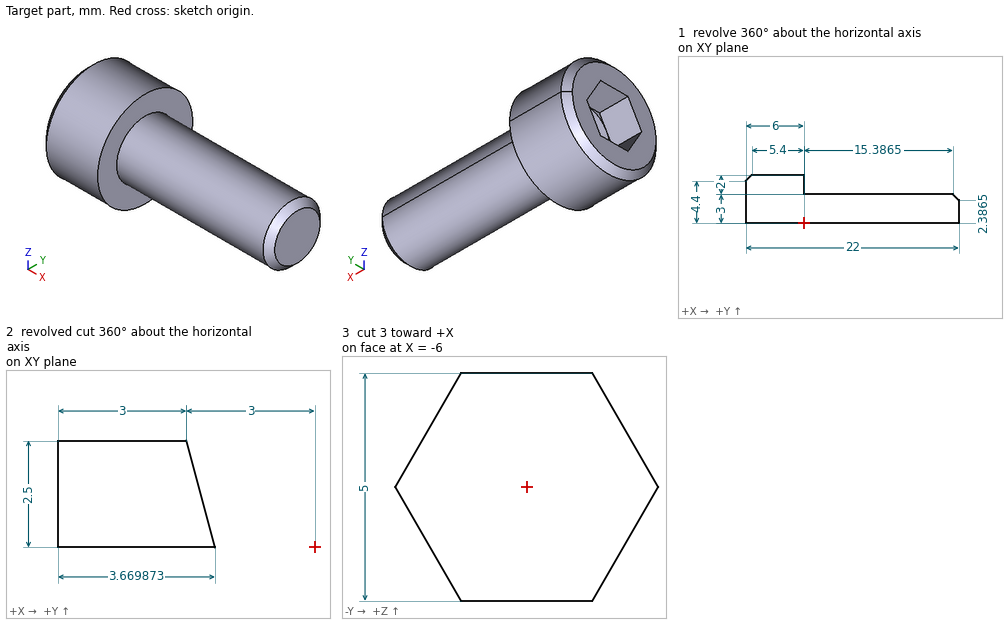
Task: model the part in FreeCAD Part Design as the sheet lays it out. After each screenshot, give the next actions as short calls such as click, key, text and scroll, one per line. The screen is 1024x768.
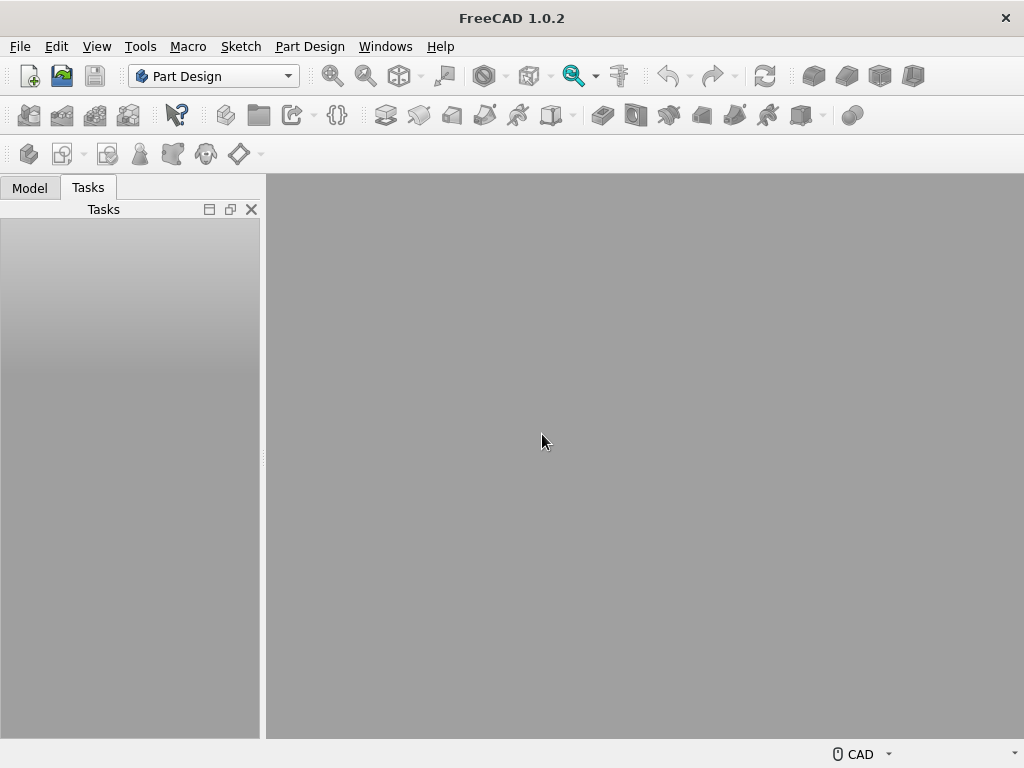
click(29, 76)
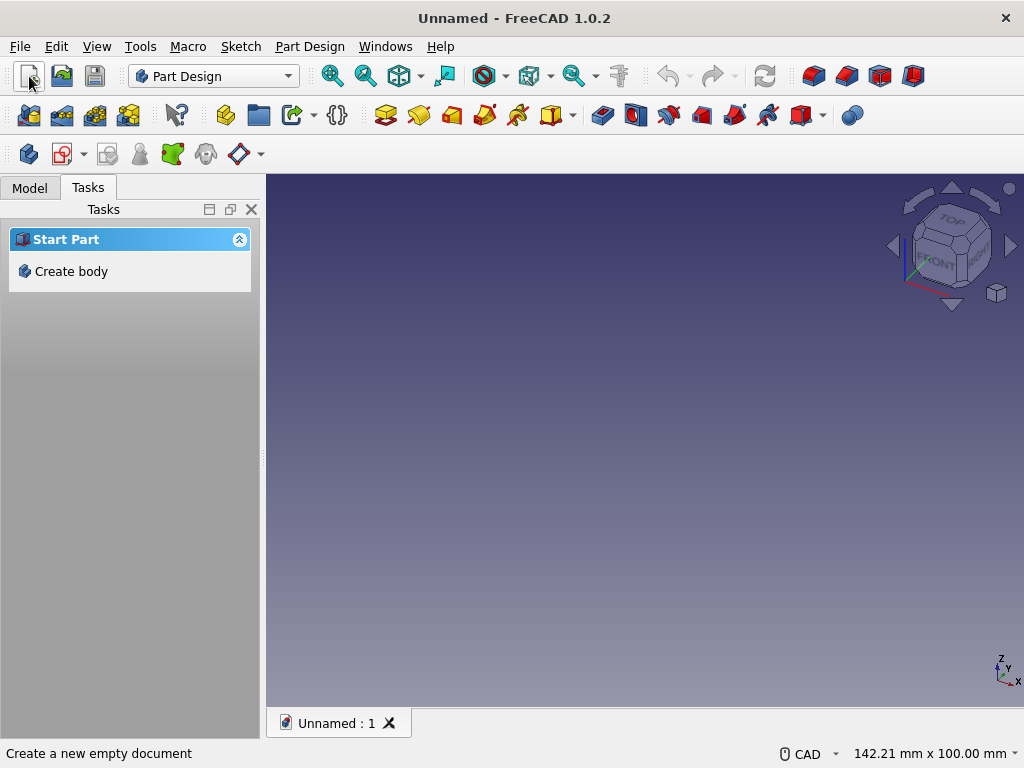
click(62, 154)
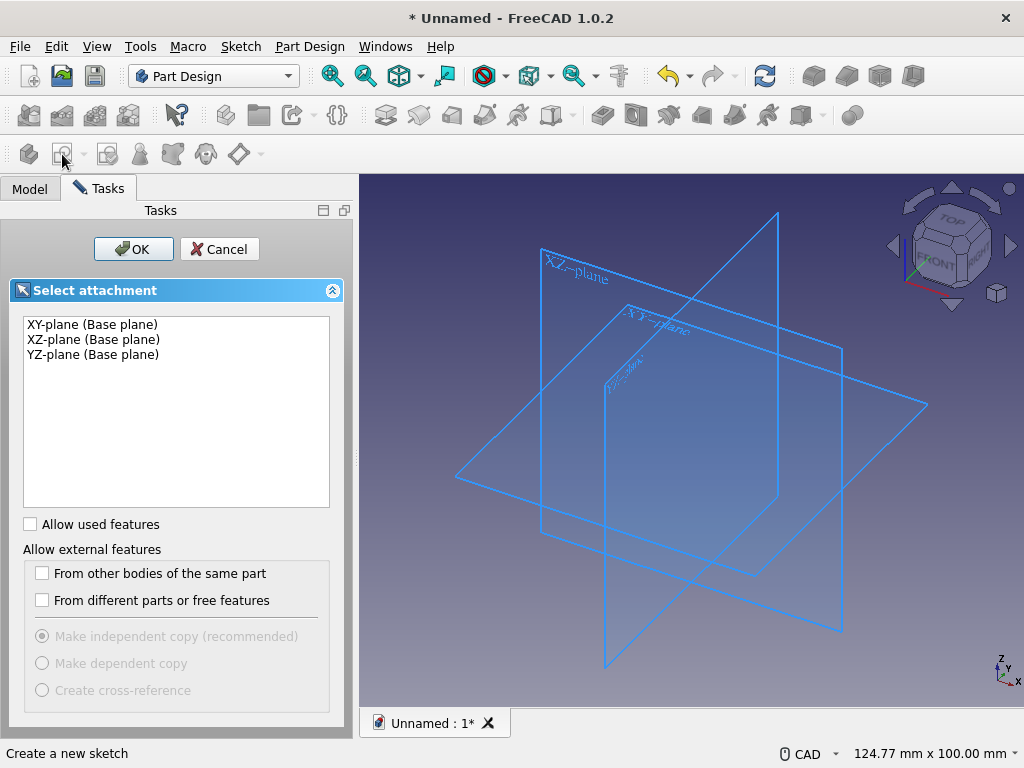
click(84, 324)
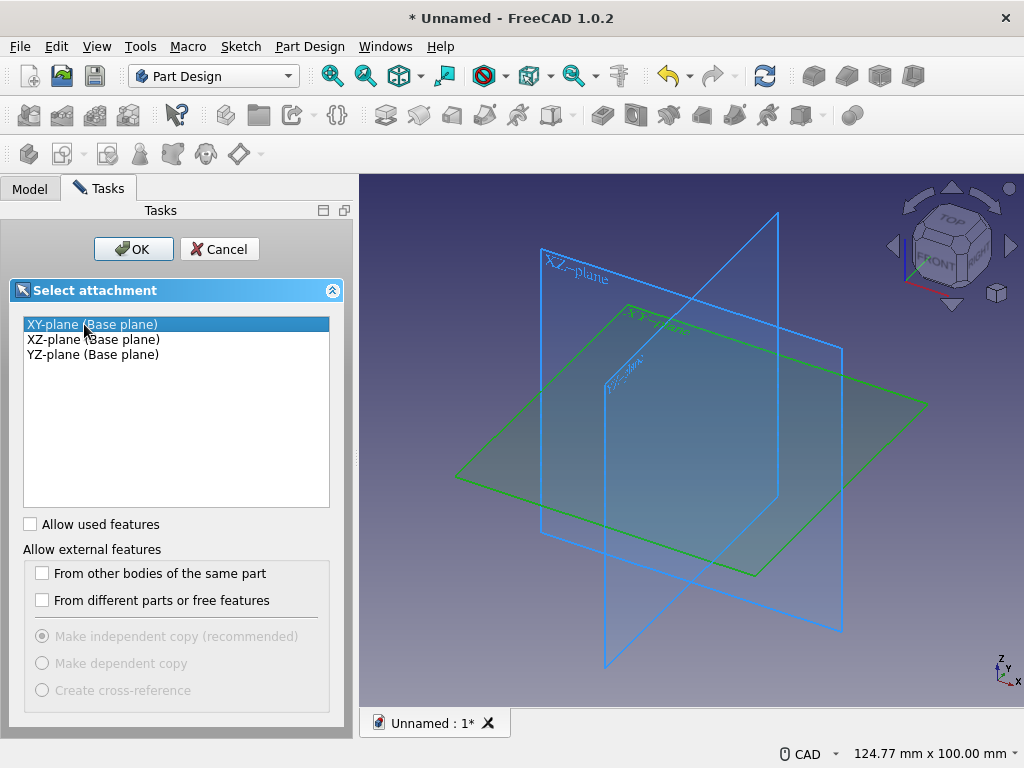
click(134, 249)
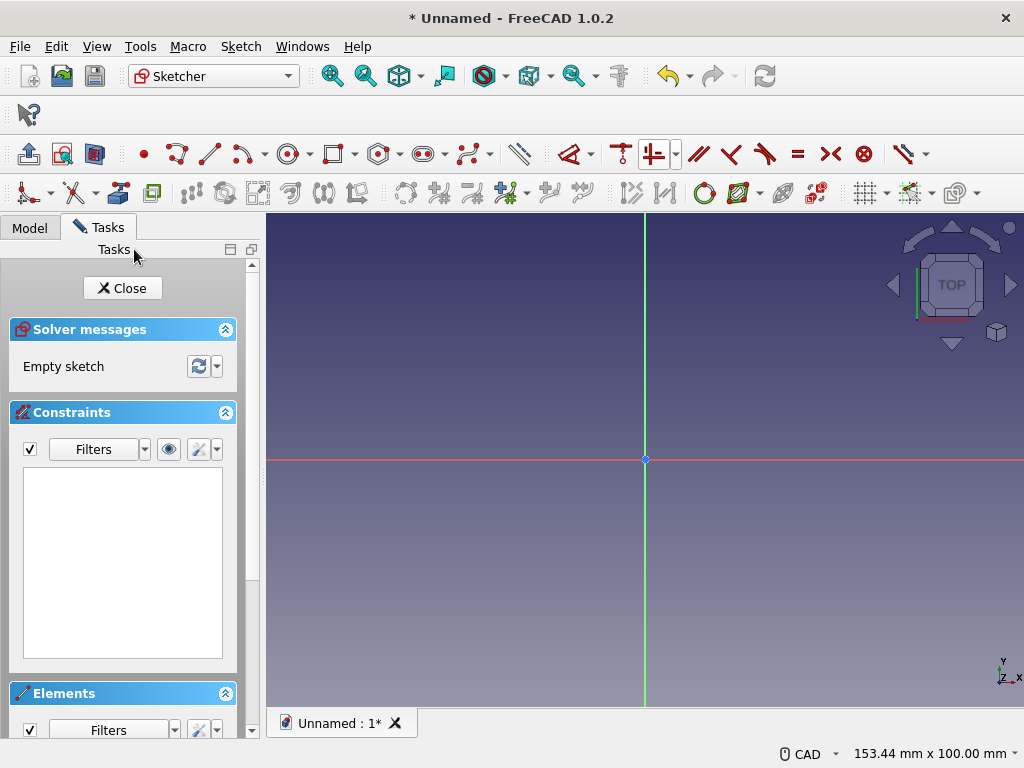
scroll(710, 442, up, 6)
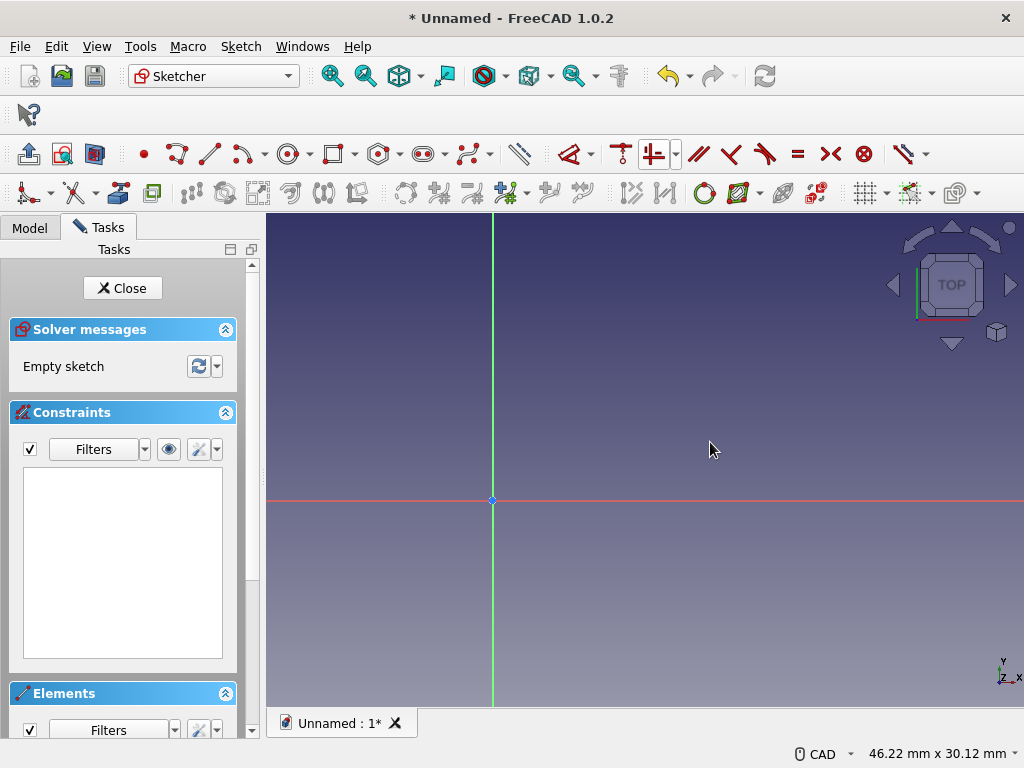
click(177, 154)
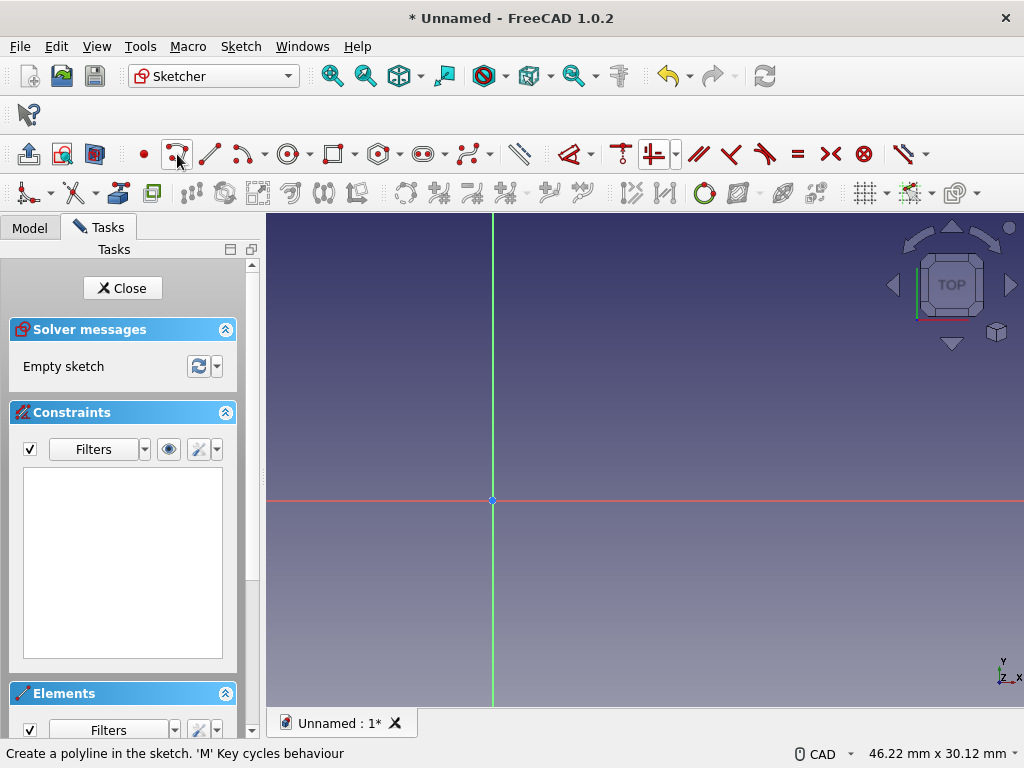
click(493, 451)
click(502, 419)
click(404, 419)
click(394, 429)
click(394, 501)
click(755, 492)
click(755, 462)
click(745, 451)
click(493, 452)
key(Escape)
key(Escape)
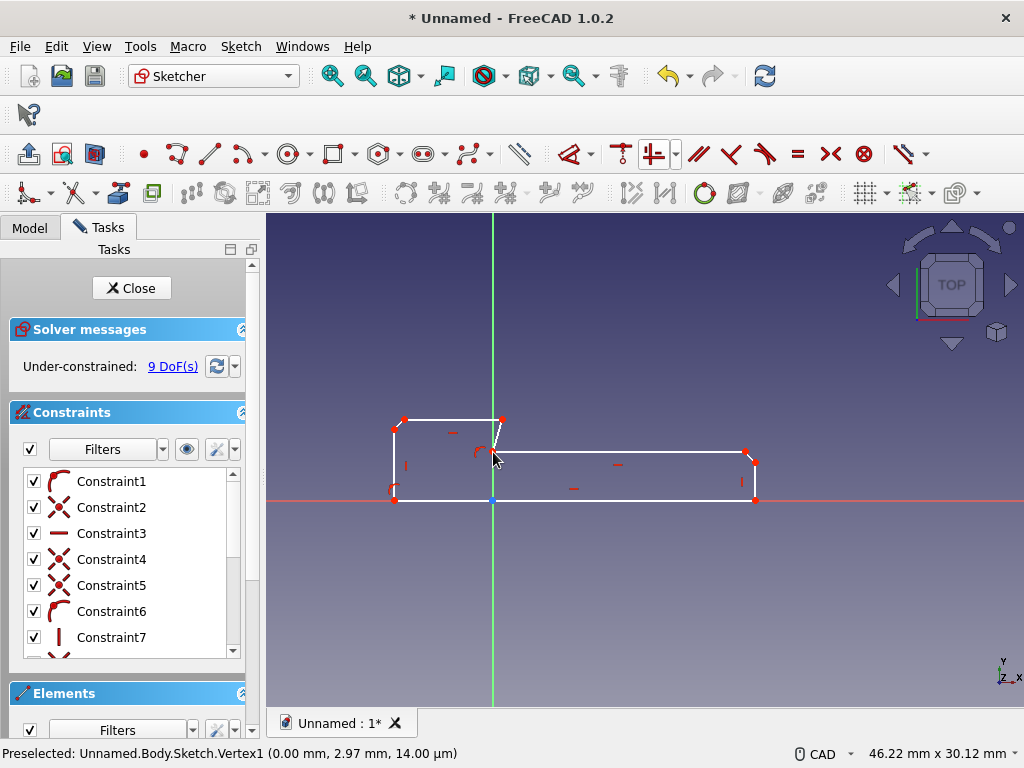
scroll(496, 442, up, 2)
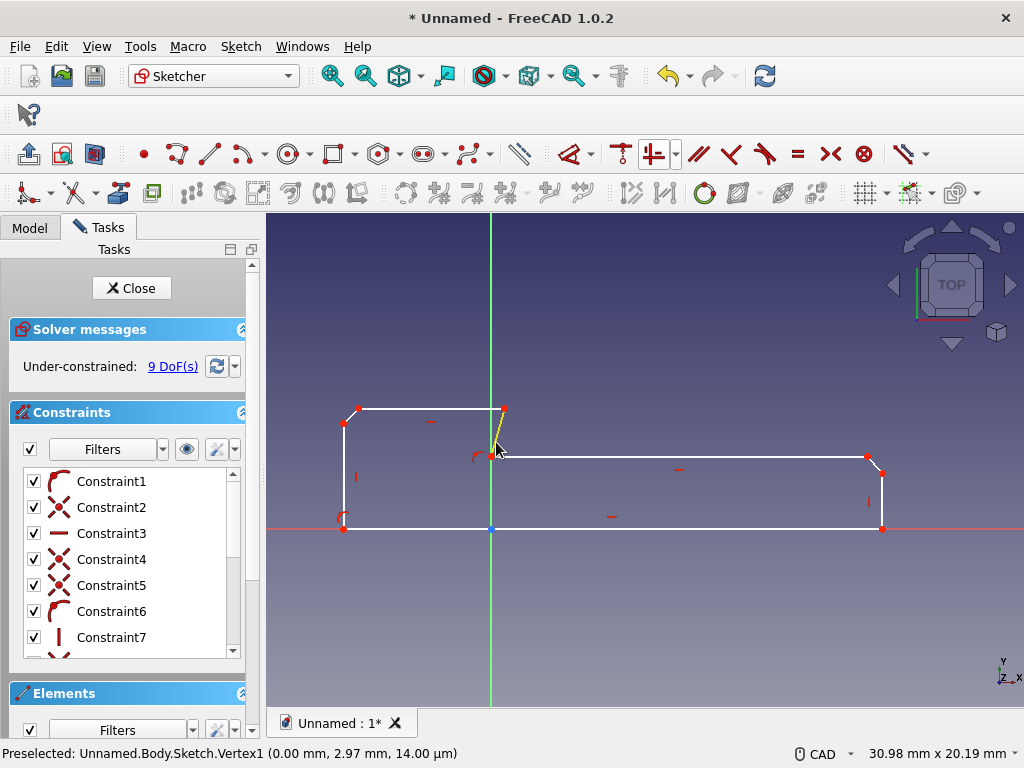
click(495, 442)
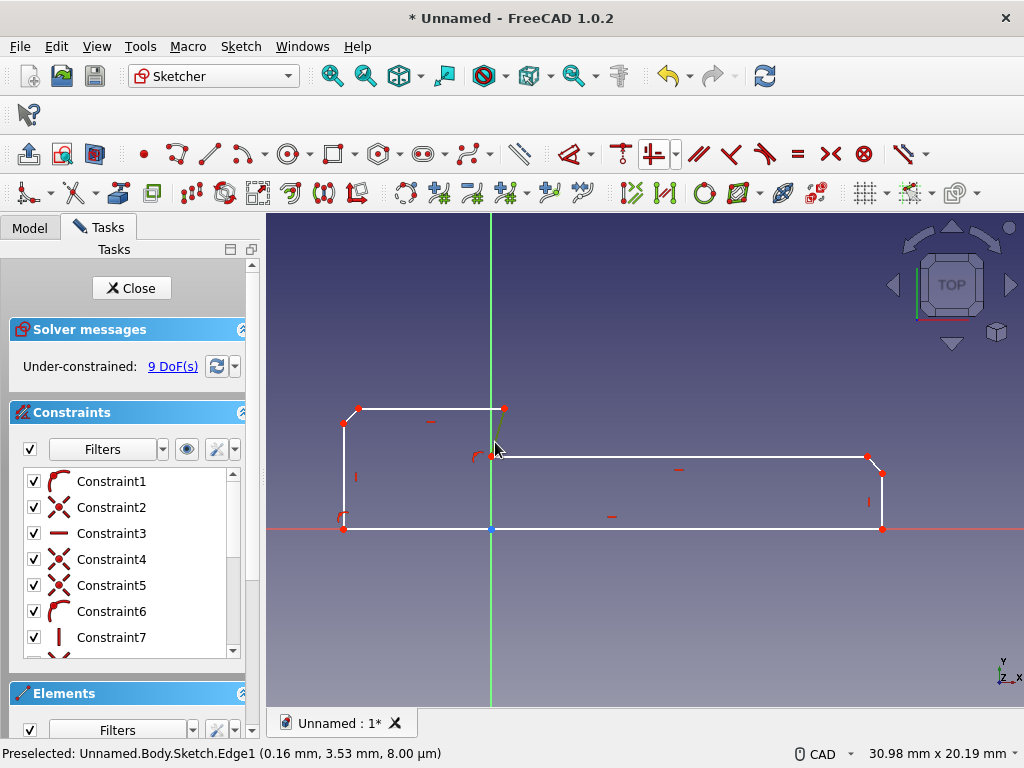
key(v)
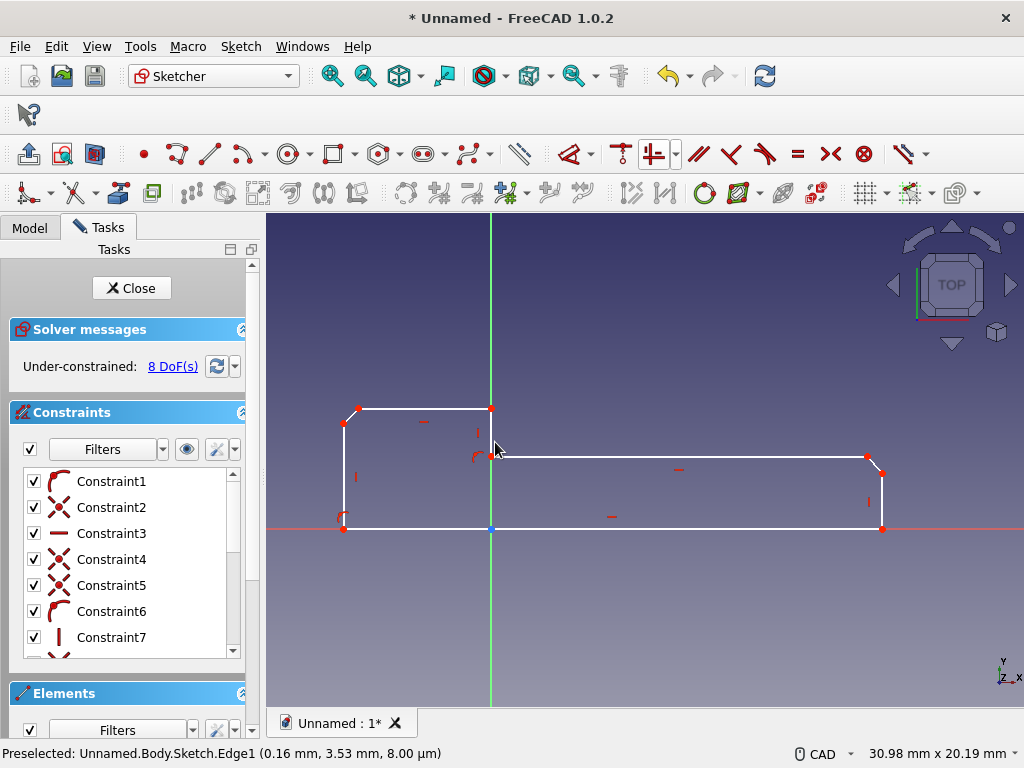
click(568, 154)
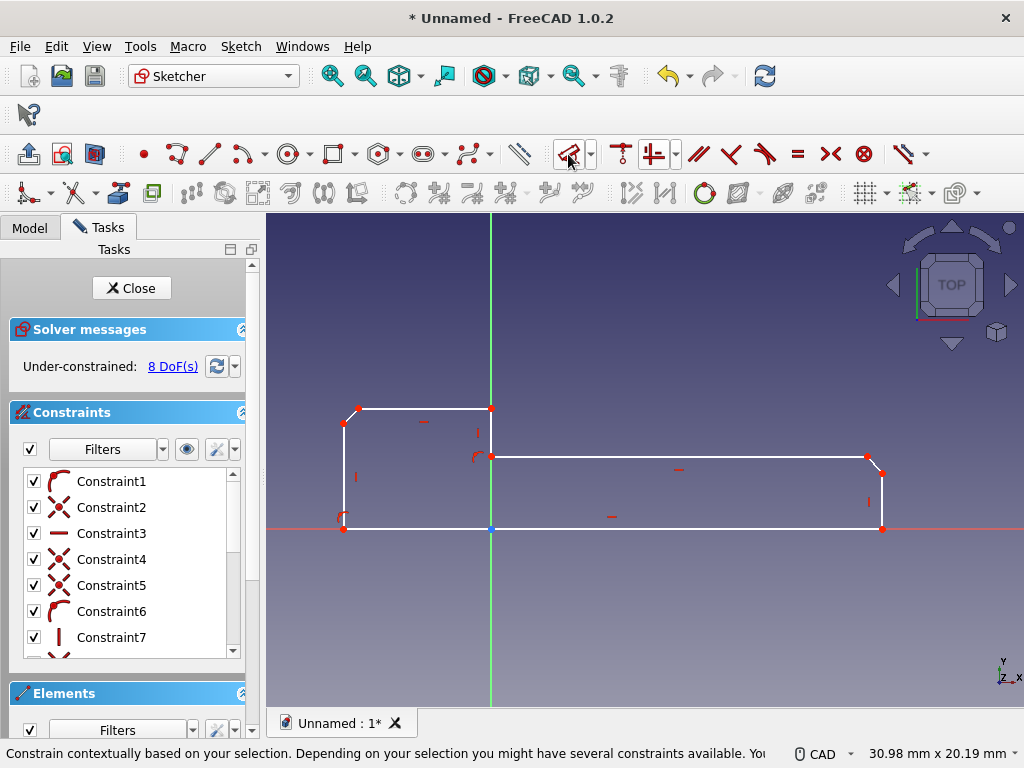
click(491, 442)
click(457, 433)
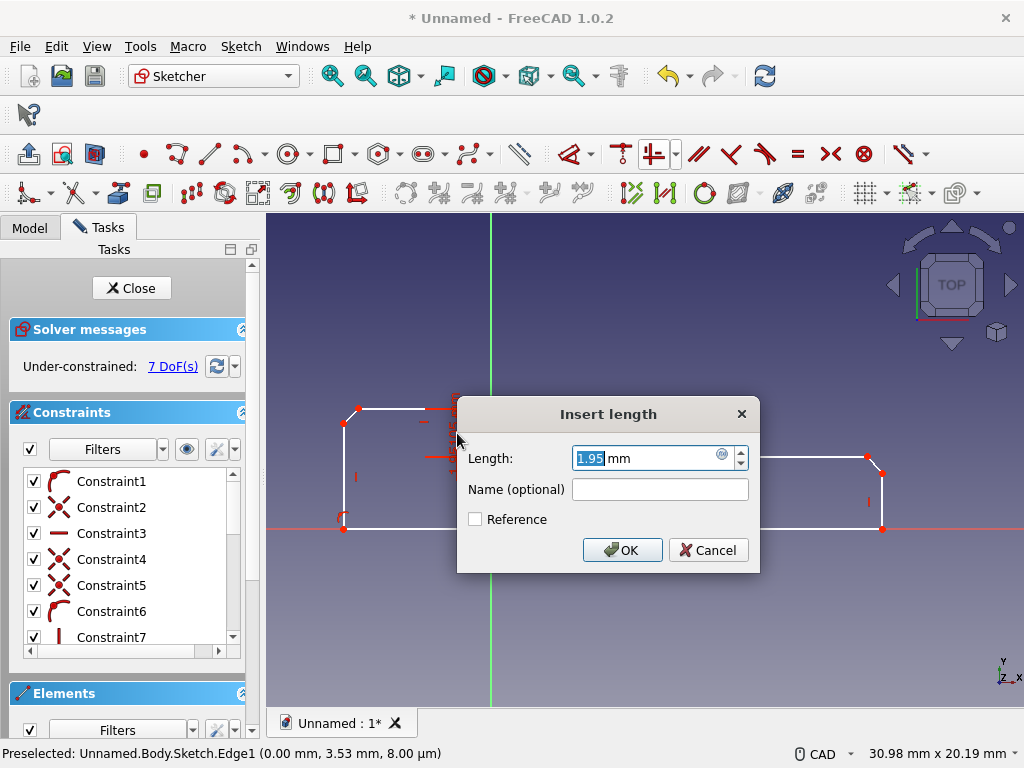
text(2)
key(Return)